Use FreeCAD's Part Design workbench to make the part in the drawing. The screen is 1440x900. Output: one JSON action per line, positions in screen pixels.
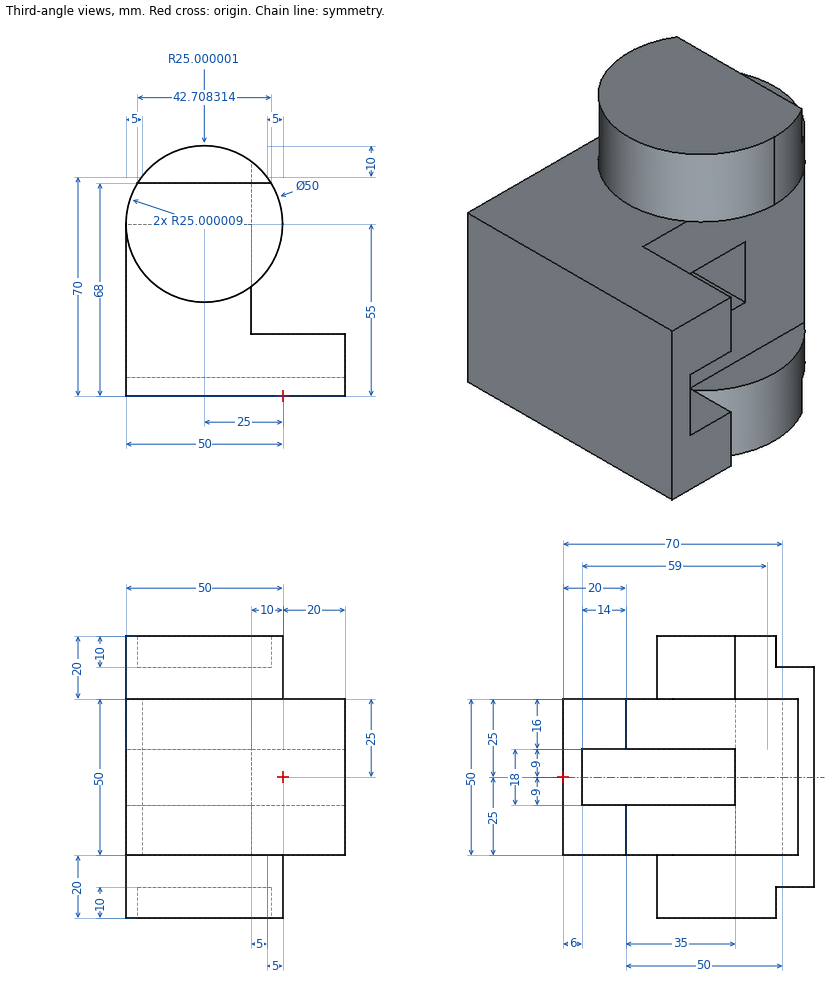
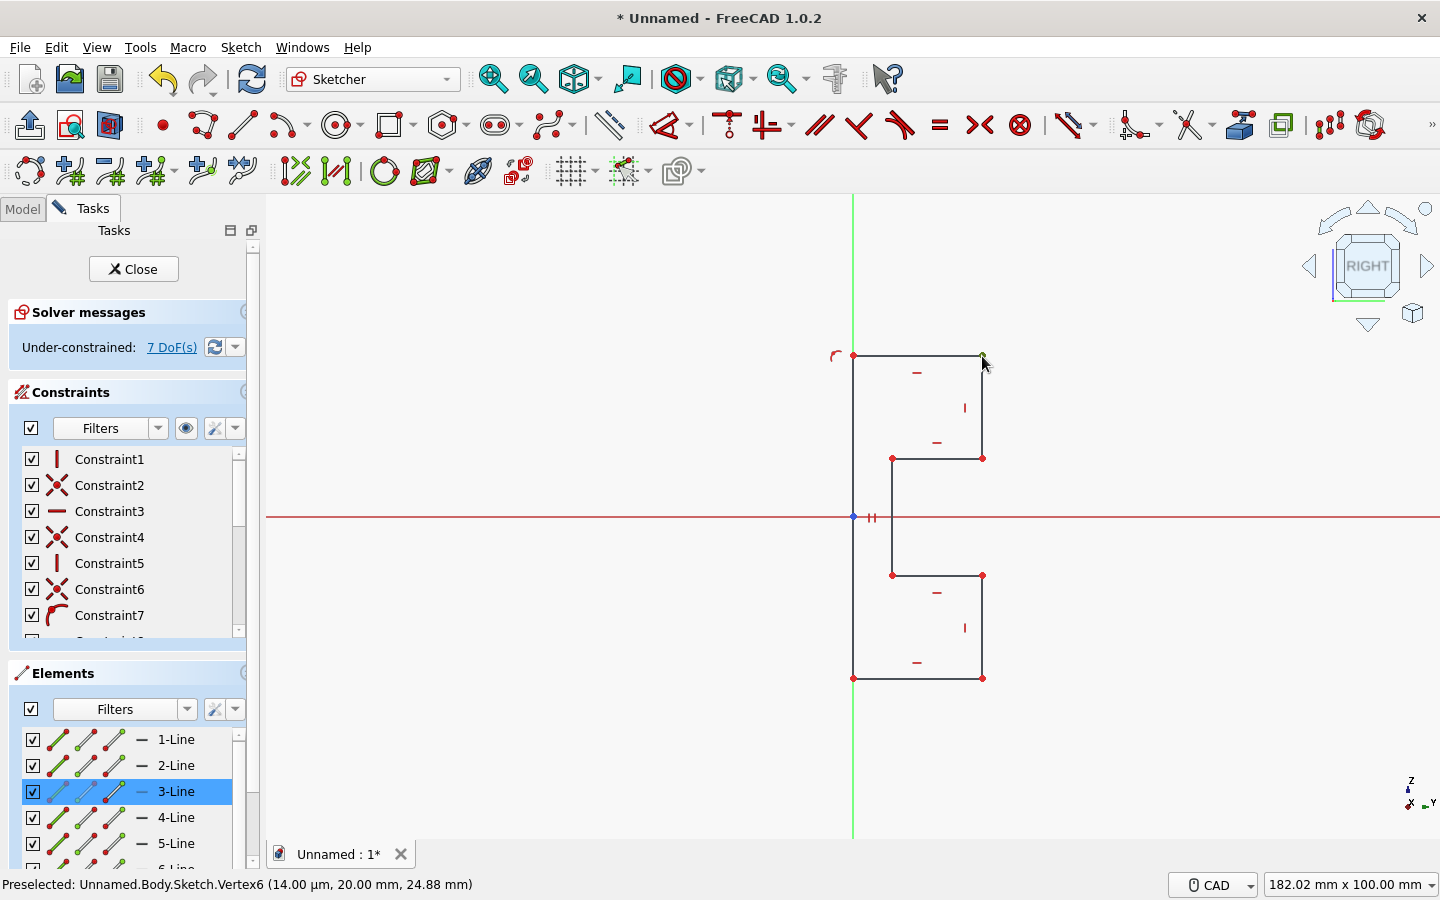
{"action": "left_click", "coordinate": [982, 679]}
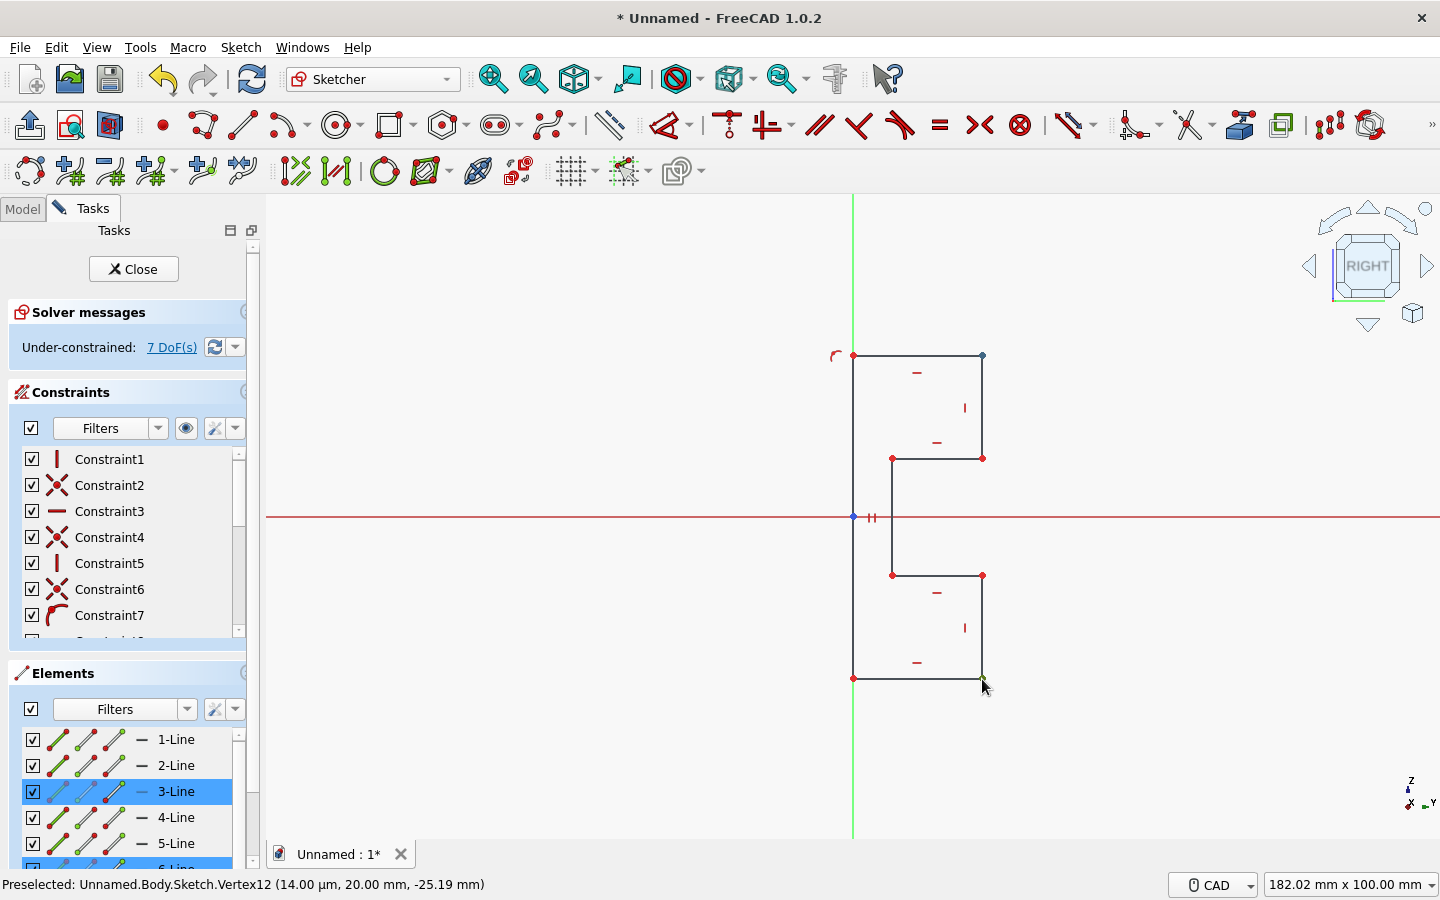
{"action": "left_click", "coordinate": [364, 516]}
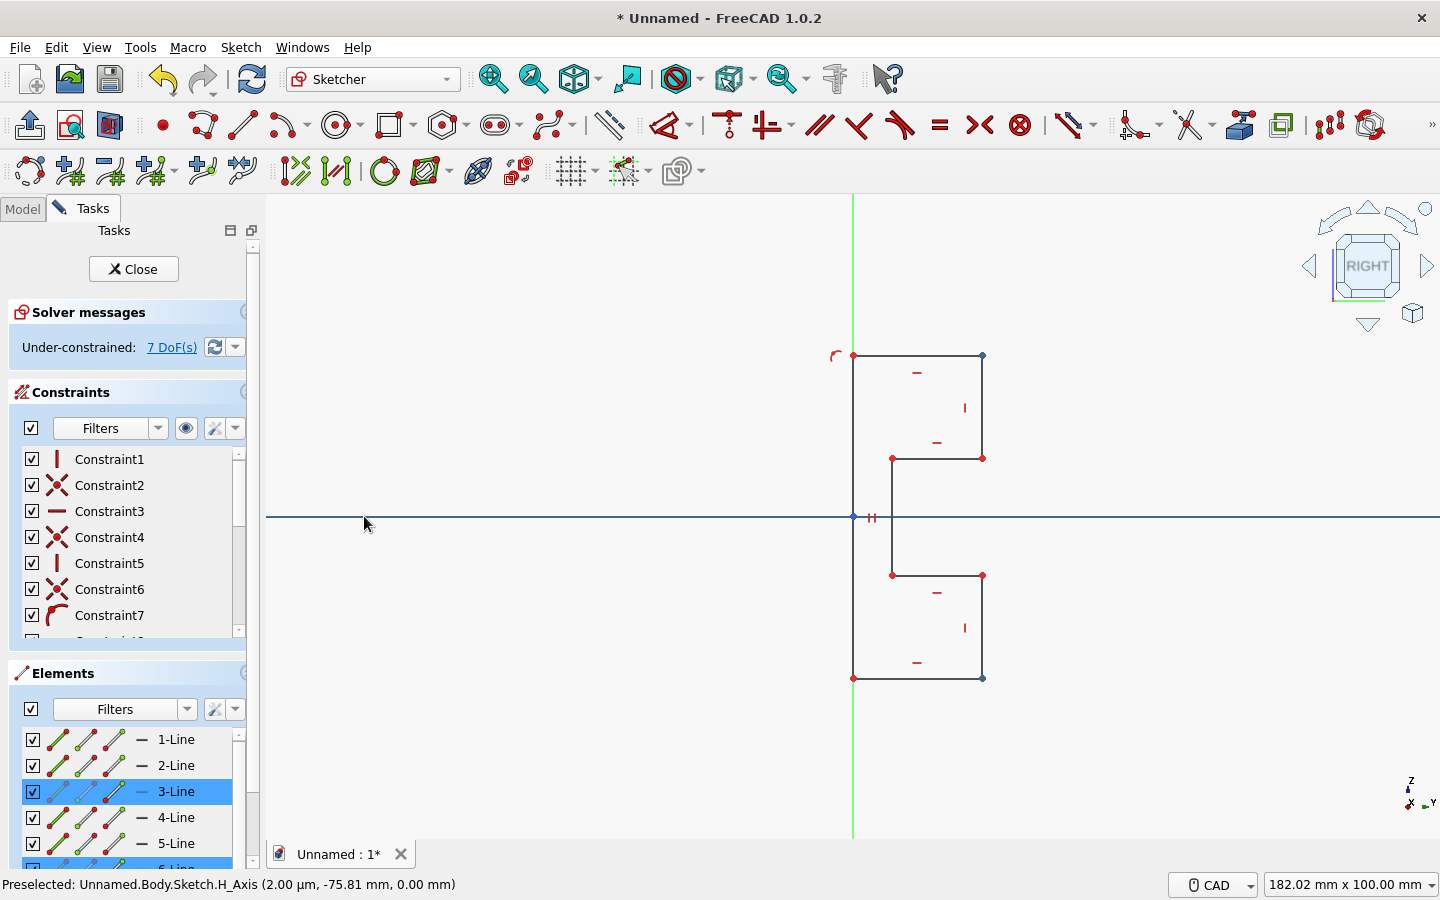
{"action": "left_click", "coordinate": [980, 126]}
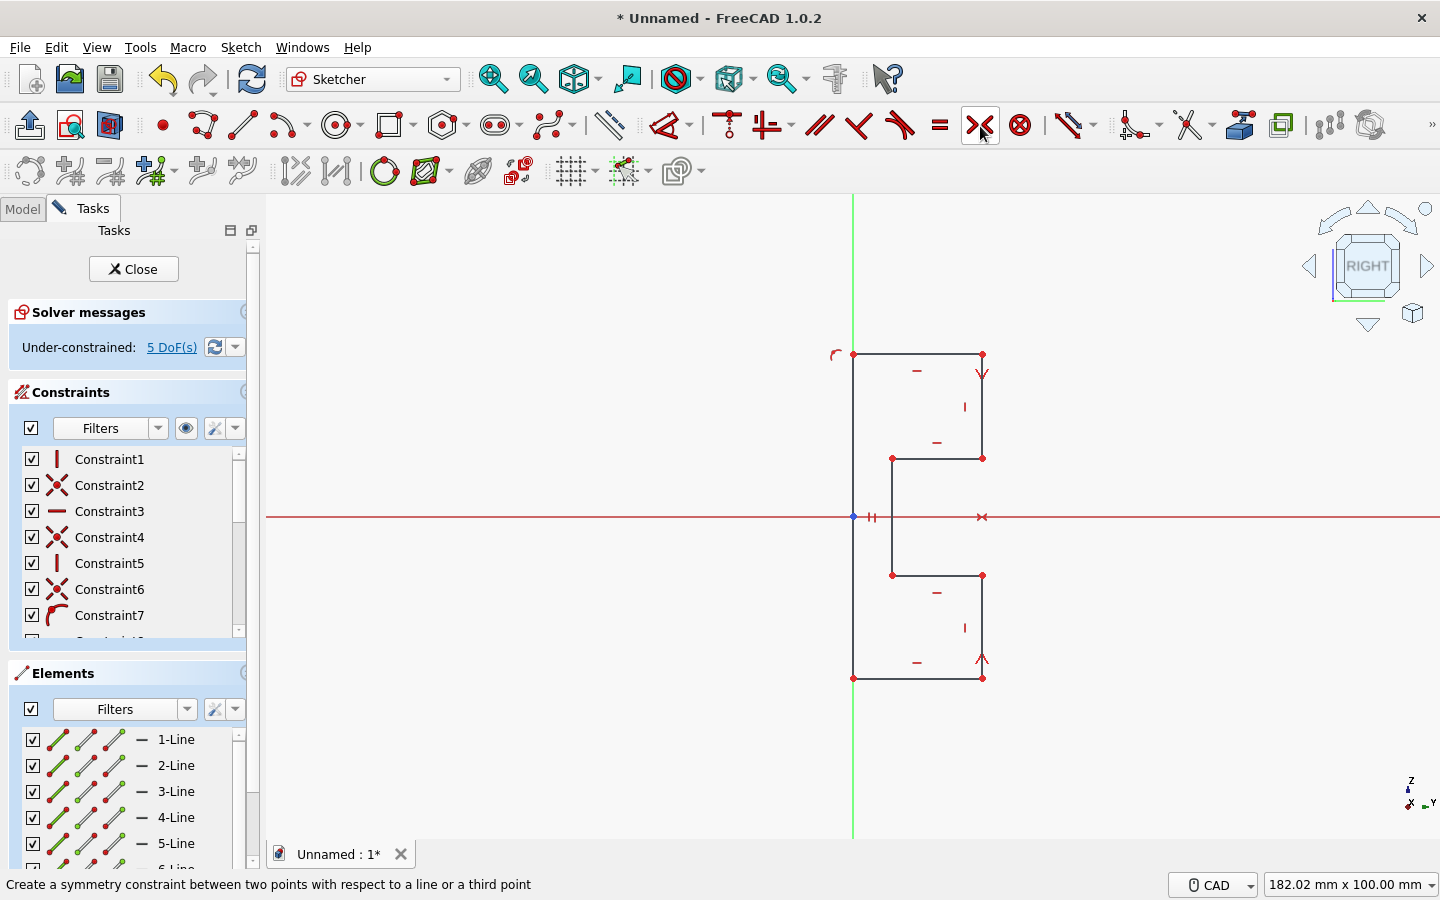
{"action": "left_click", "coordinate": [664, 126]}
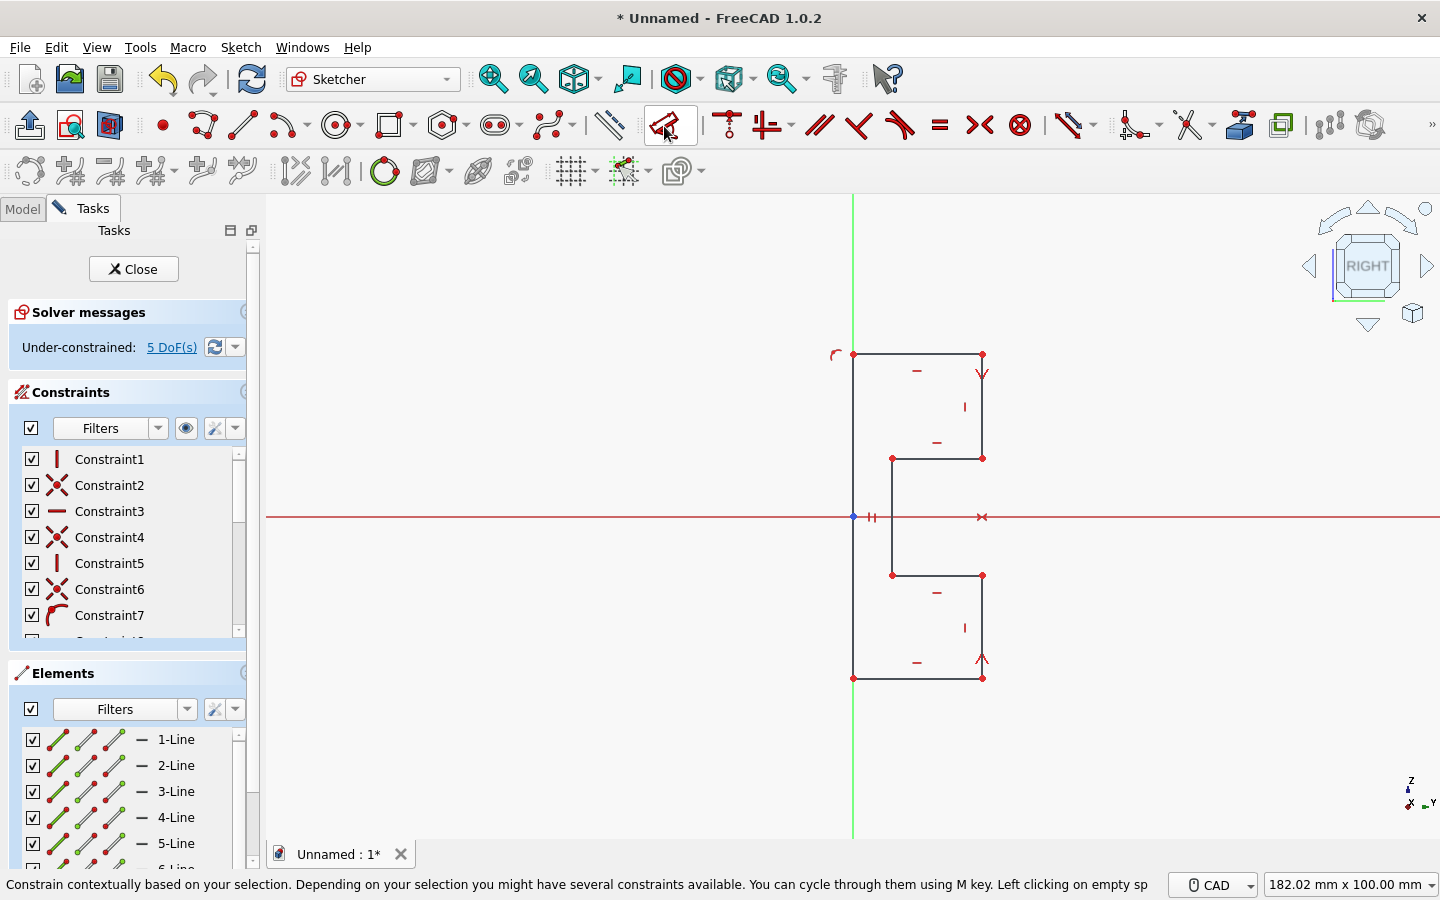
{"action": "left_click", "coordinate": [892, 541]}
{"action": "left_click", "coordinate": [926, 491]}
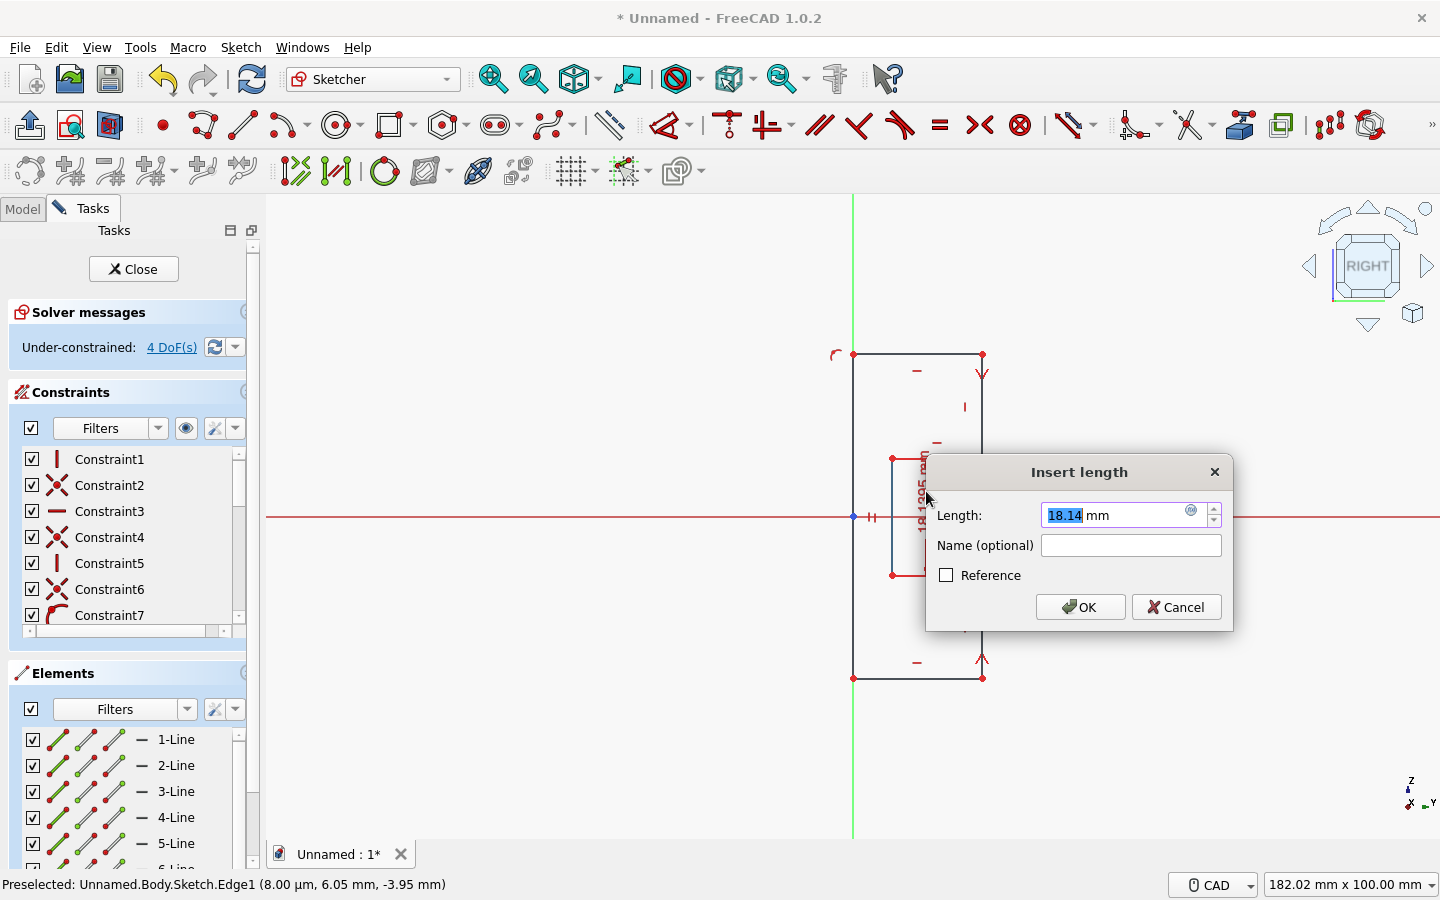
{"action": "type", "text": "18"}
{"action": "key", "text": "Return"}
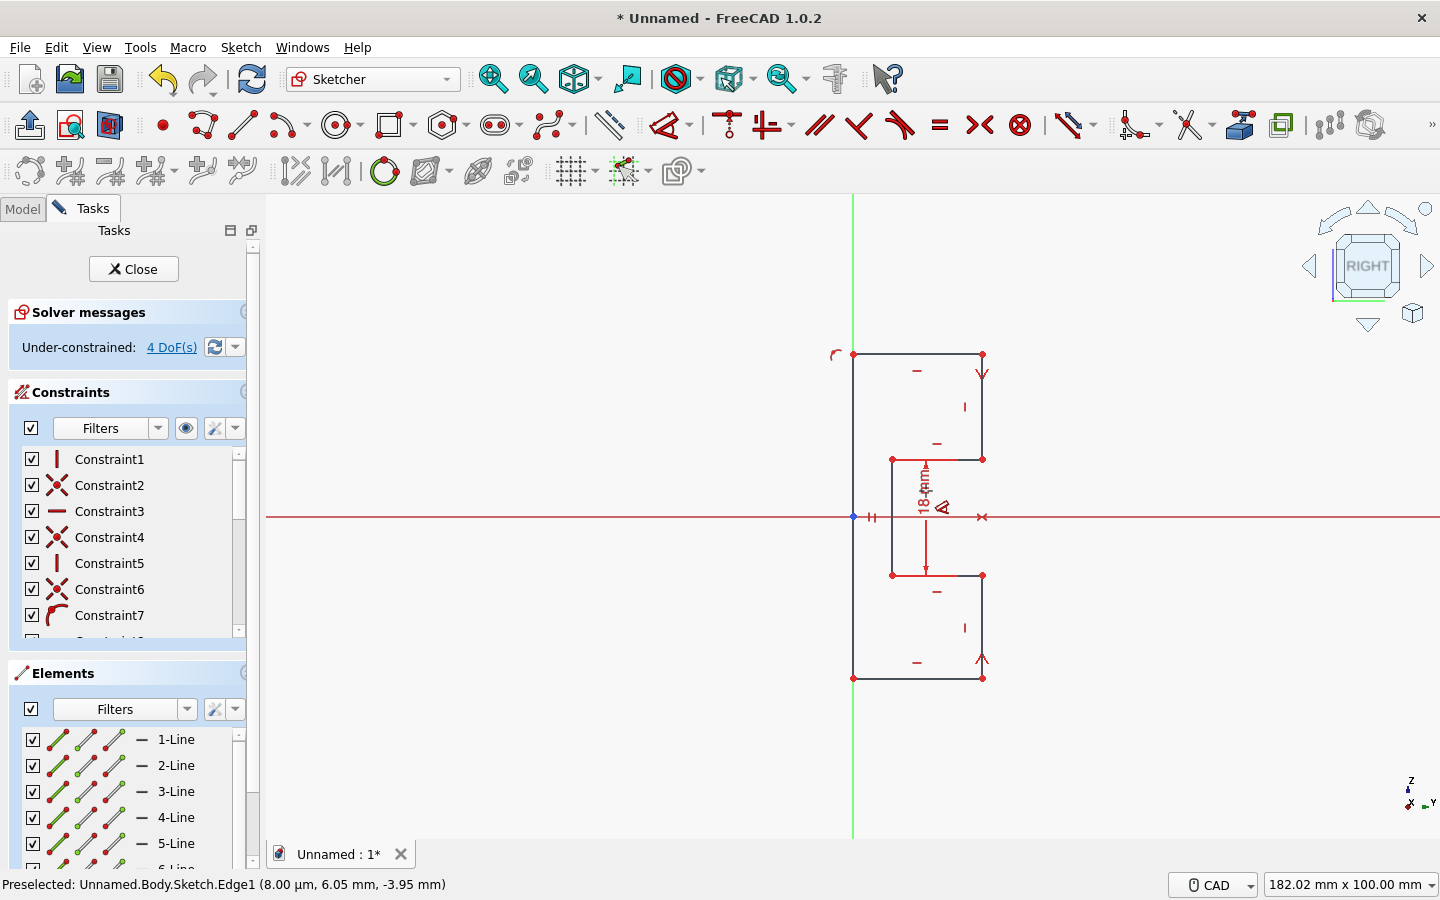
{"action": "left_click", "coordinate": [919, 460]}
{"action": "left_click", "coordinate": [937, 426]}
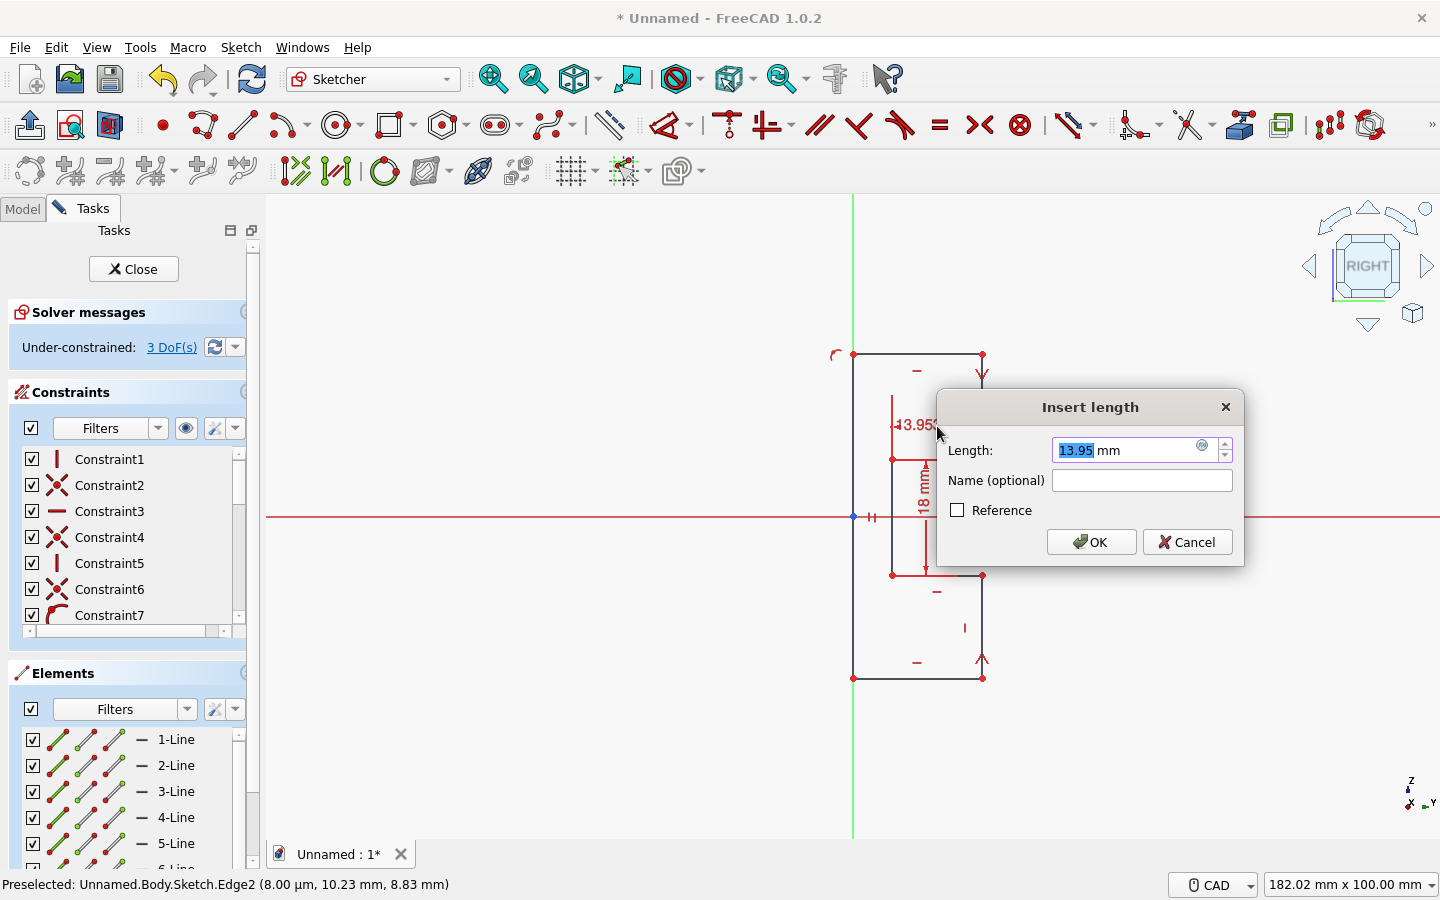
{"action": "type", "text": "14"}
{"action": "key", "text": "Return"}